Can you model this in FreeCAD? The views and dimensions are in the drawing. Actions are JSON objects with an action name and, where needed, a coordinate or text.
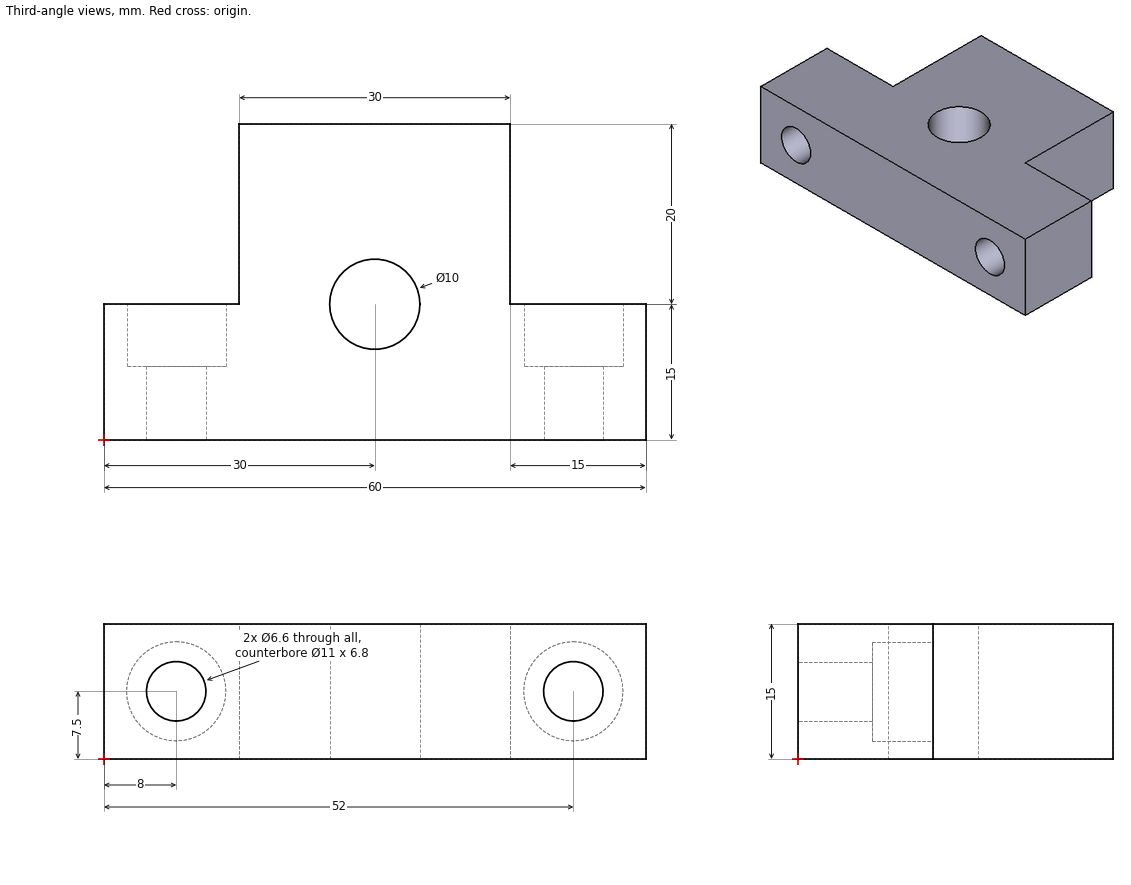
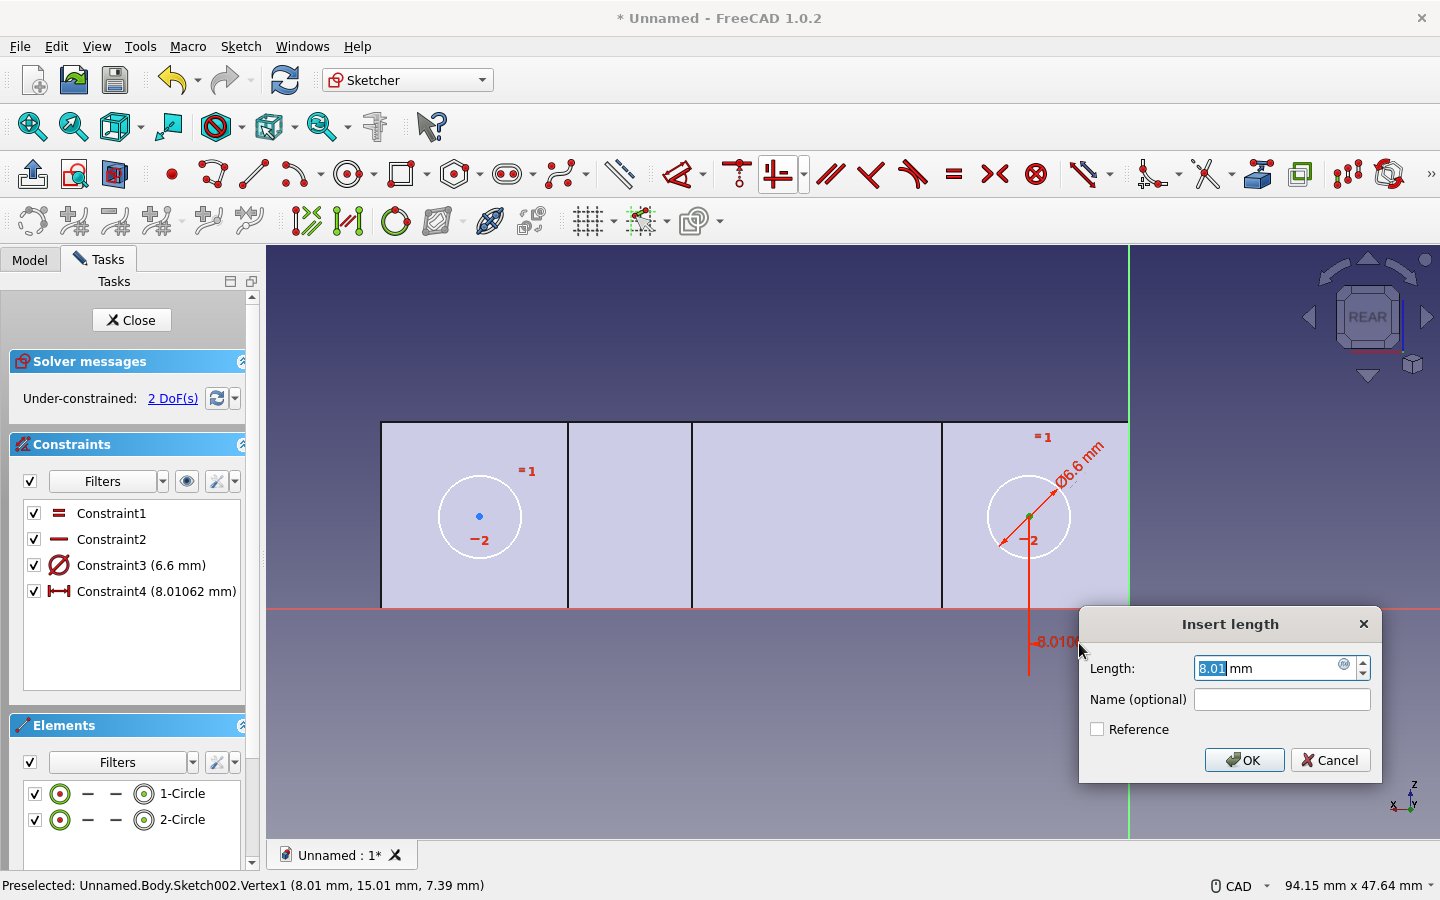
{"action": "type", "text": "8"}
{"action": "key", "text": "Return"}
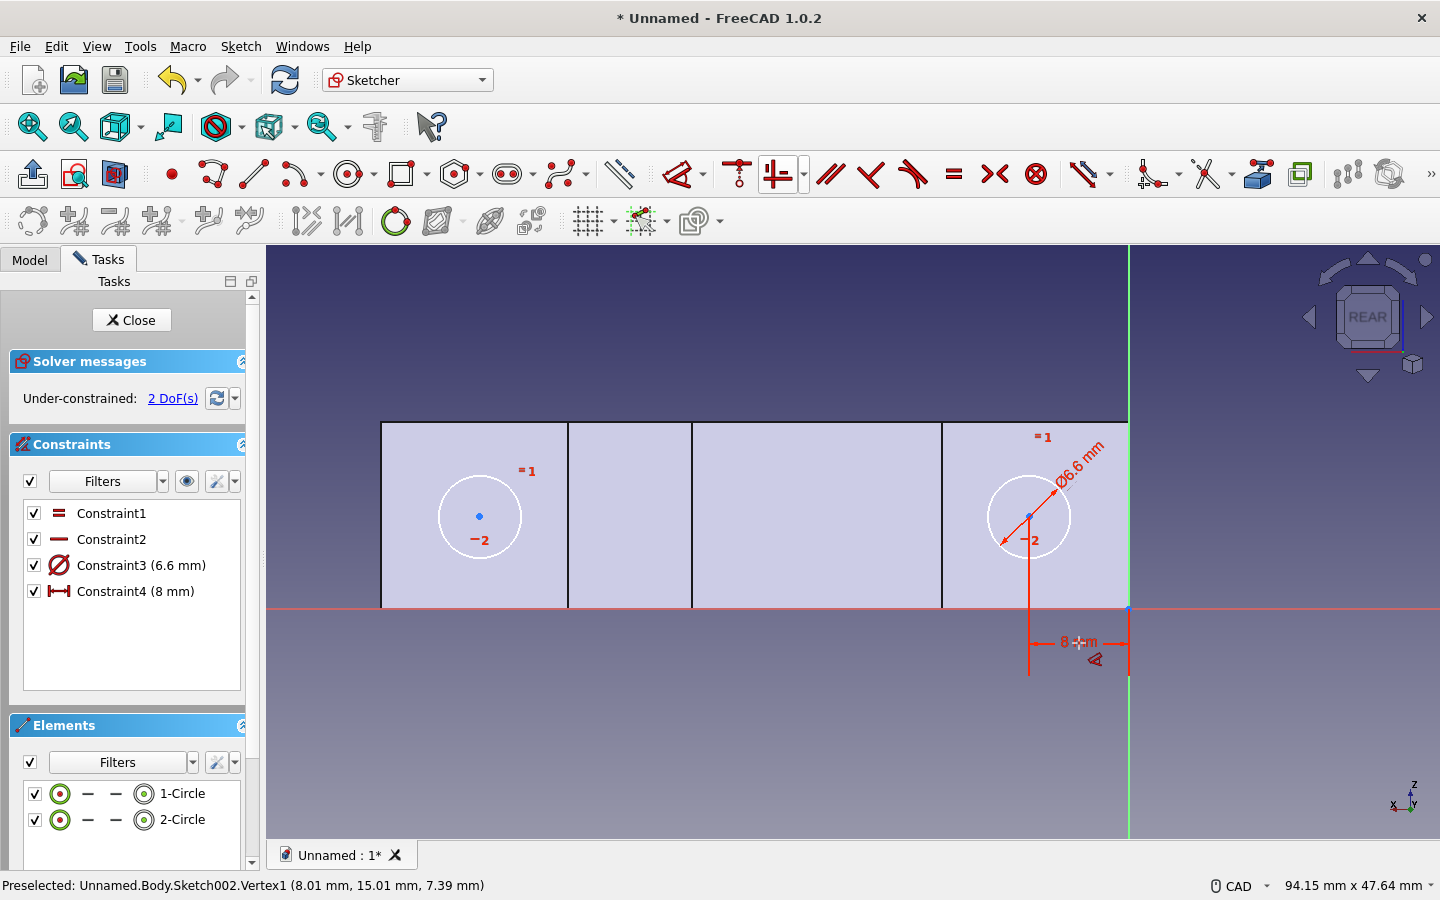
{"action": "left_click", "coordinate": [480, 517]}
{"action": "left_click", "coordinate": [804, 643]}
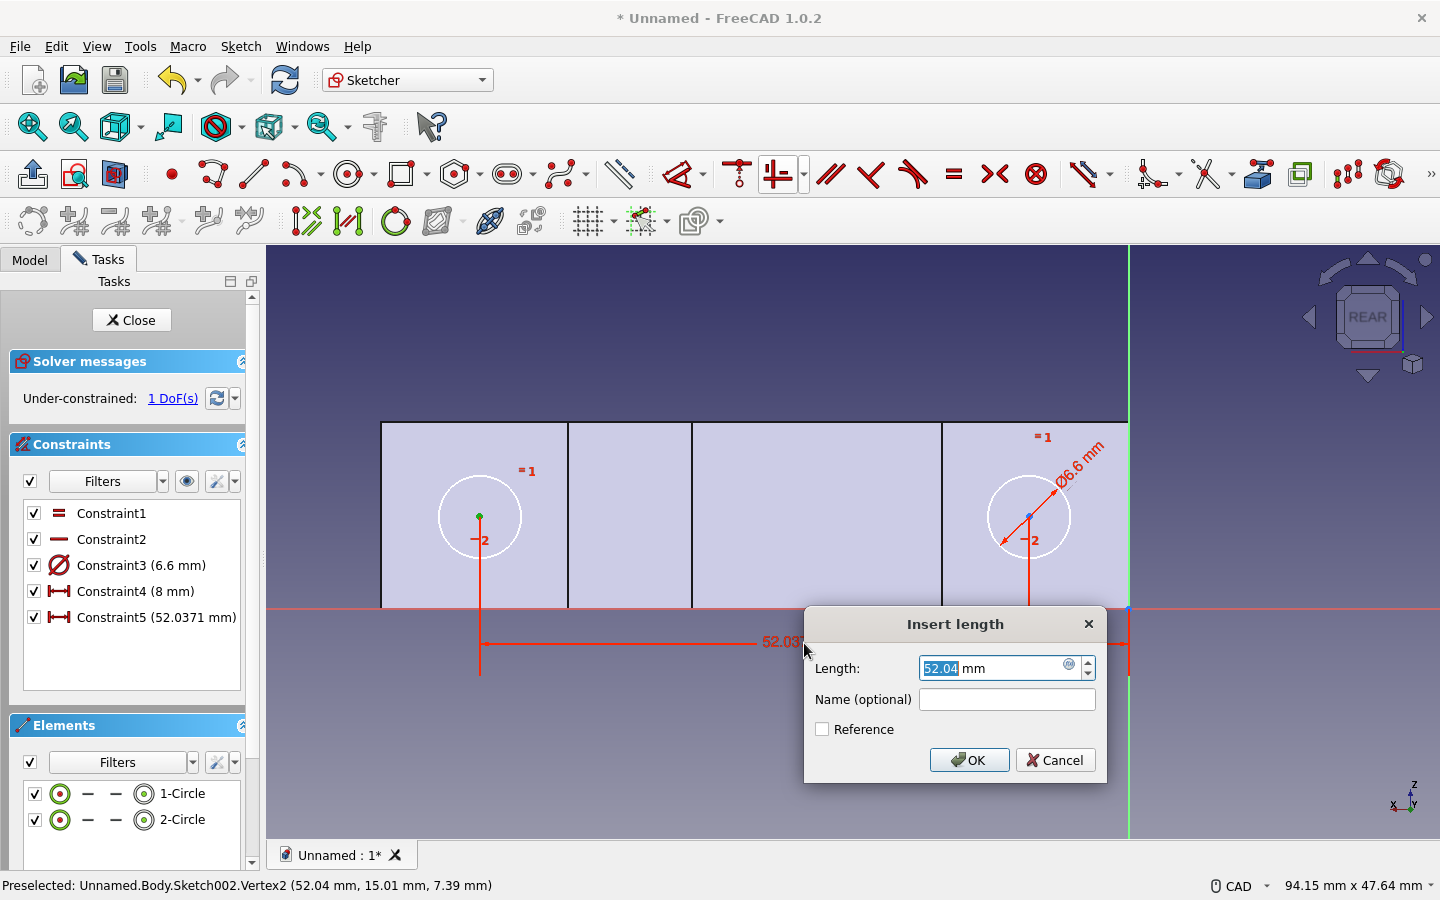
{"action": "type", "text": "52"}
{"action": "key", "text": "Return"}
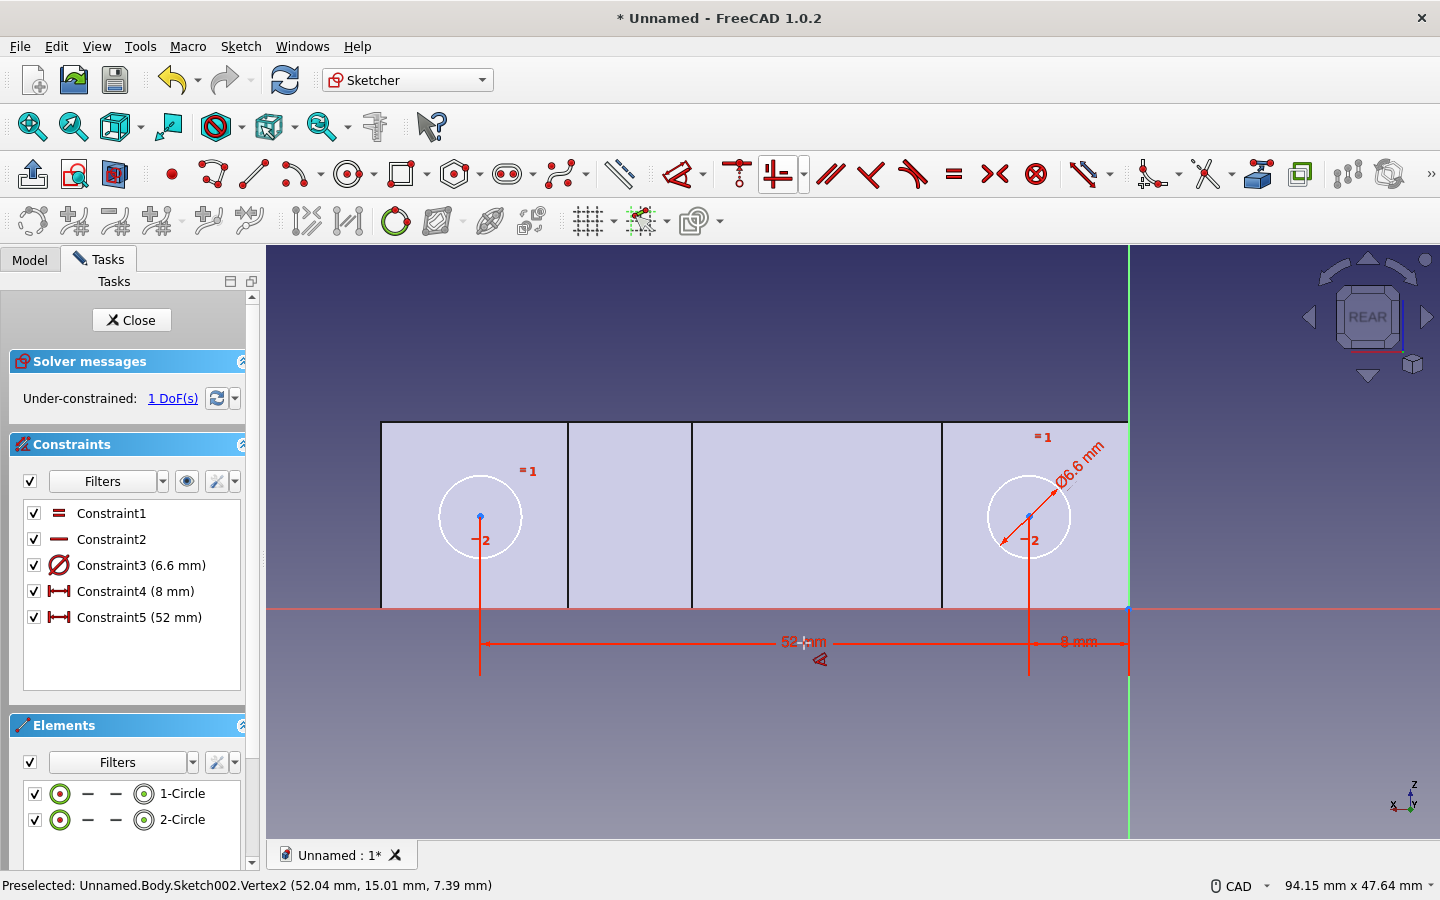
{"action": "left_click", "coordinate": [1029, 517]}
{"action": "left_click", "coordinate": [1163, 563]}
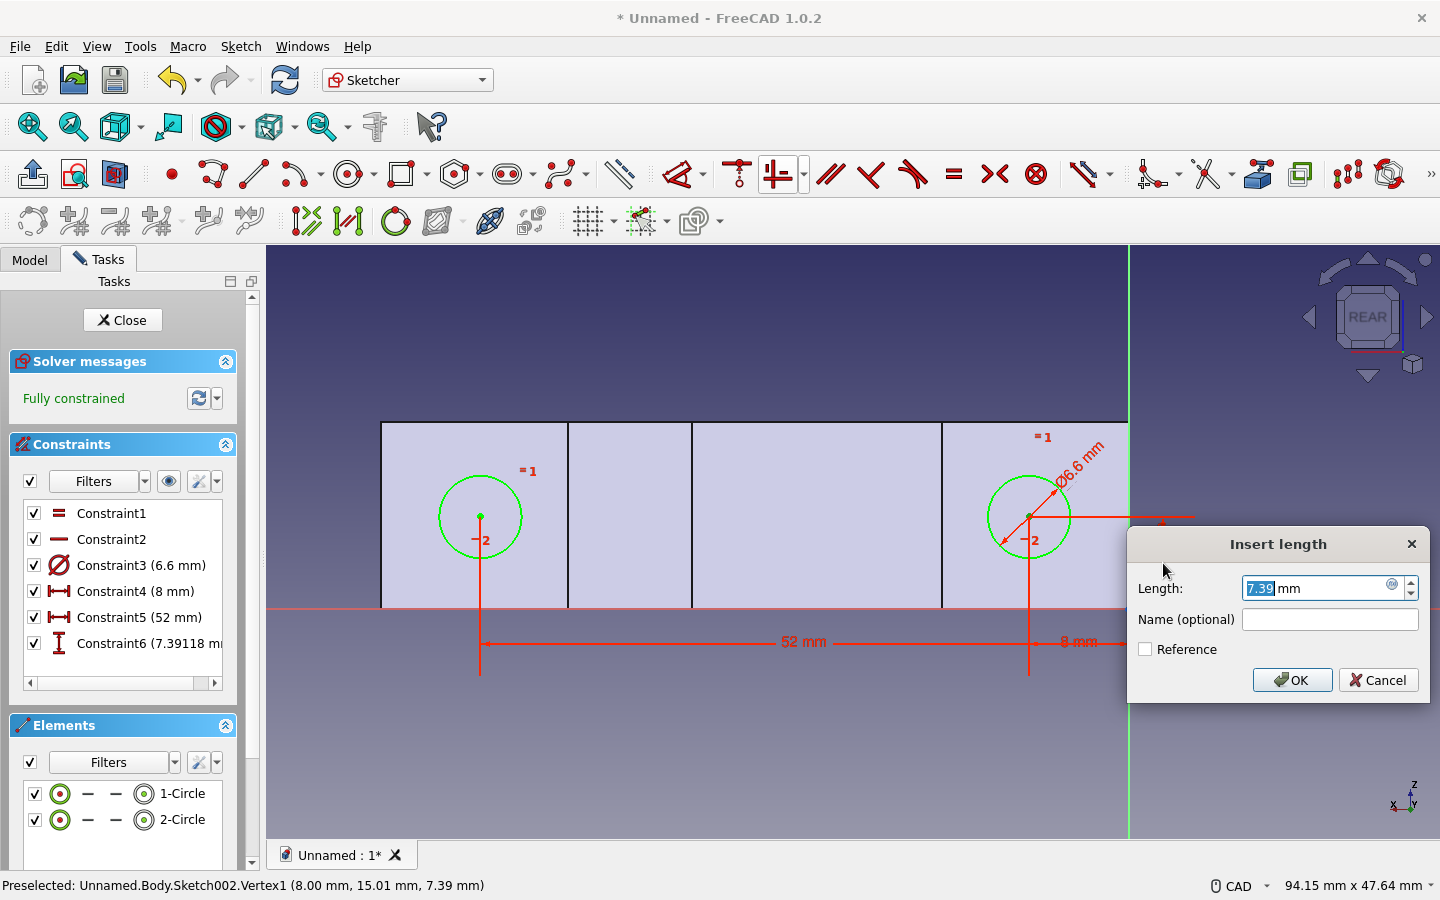
{"action": "type", "text": "7.5"}
{"action": "key", "text": "Return"}
{"action": "key", "text": "Escape"}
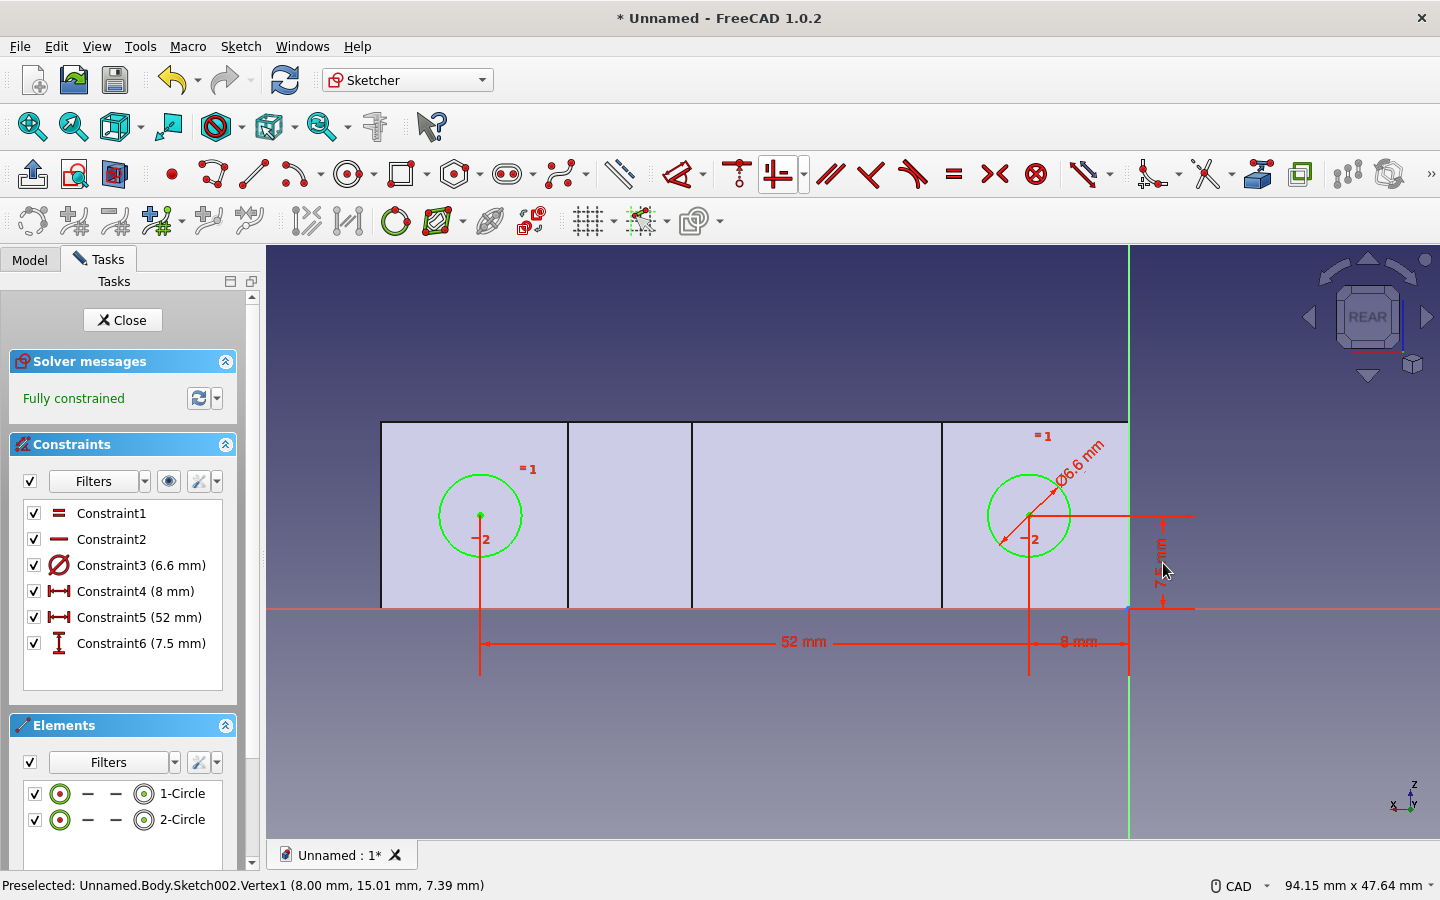
{"action": "left_click", "coordinate": [123, 320]}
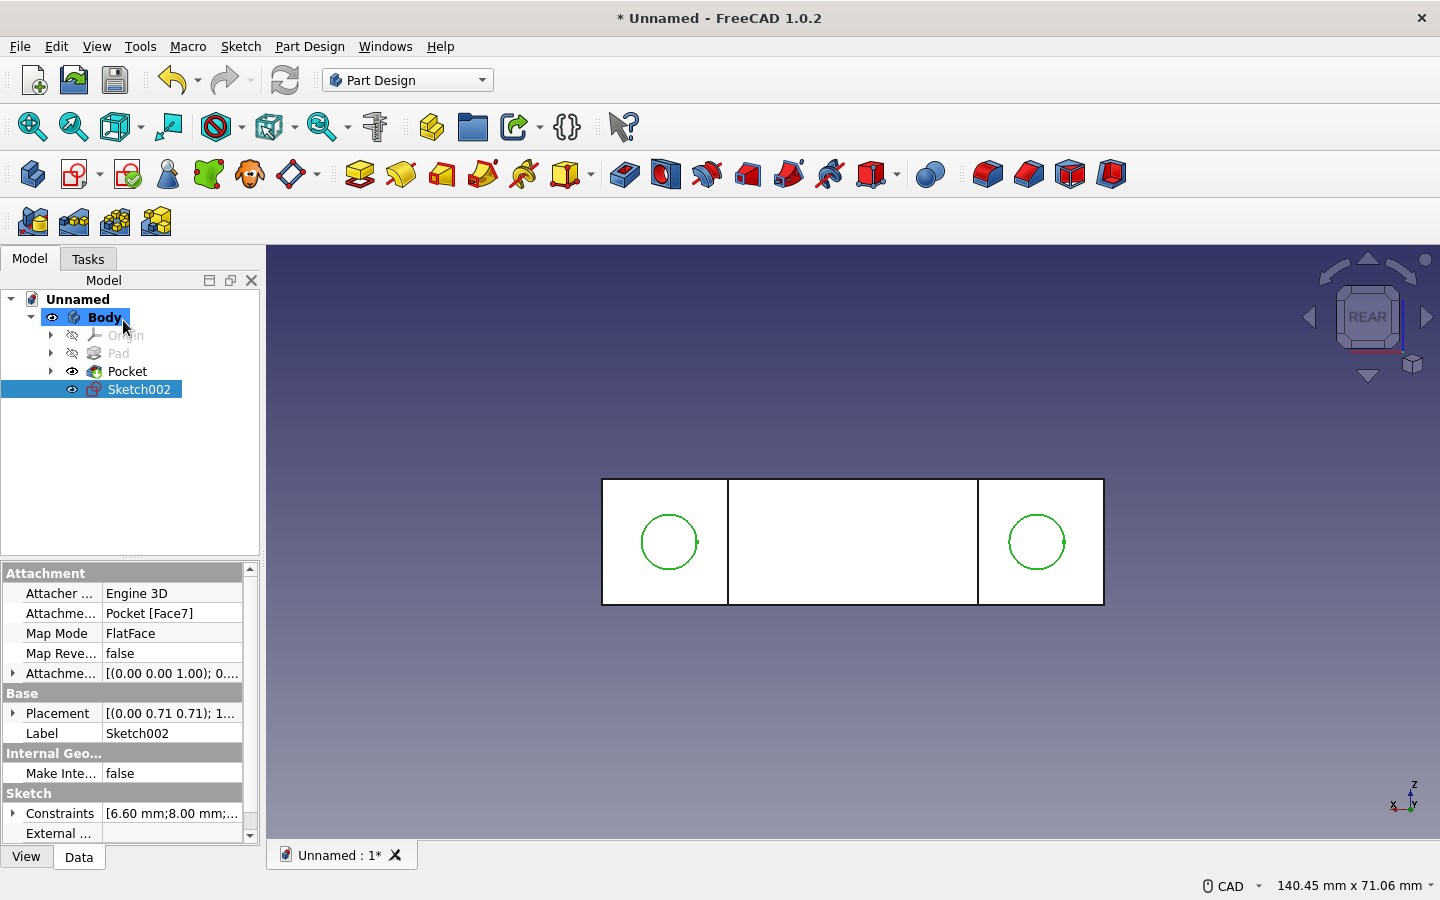
{"action": "left_click", "coordinate": [666, 174]}